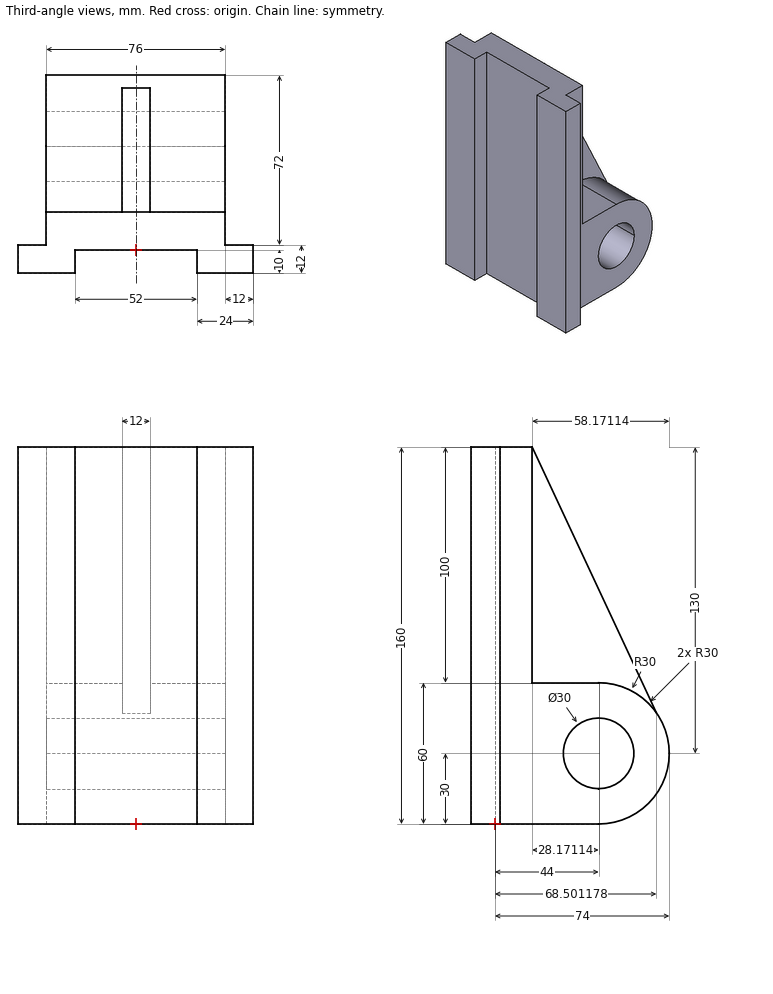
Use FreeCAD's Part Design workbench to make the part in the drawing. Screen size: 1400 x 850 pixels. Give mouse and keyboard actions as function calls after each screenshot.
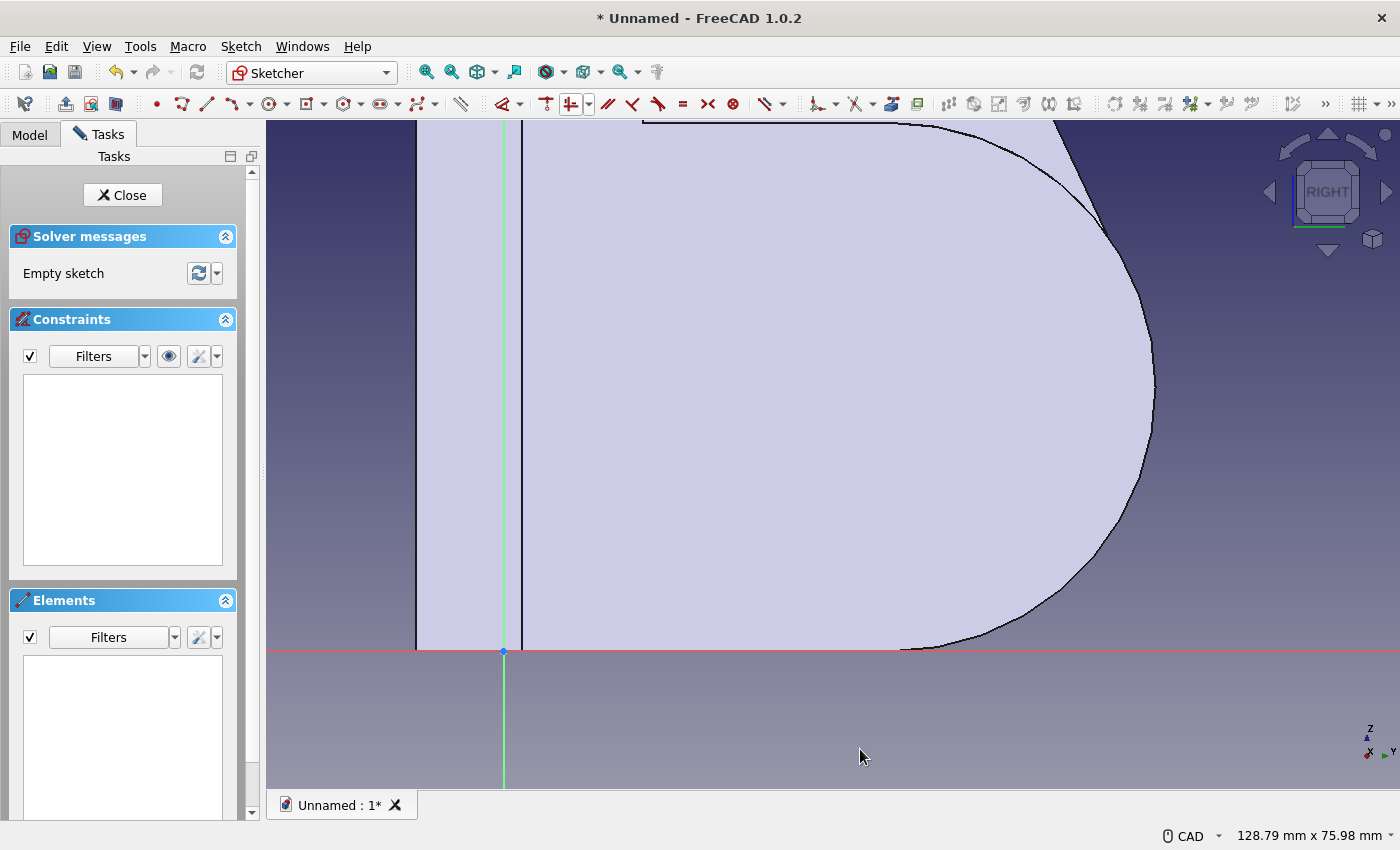
key(g)
key(c)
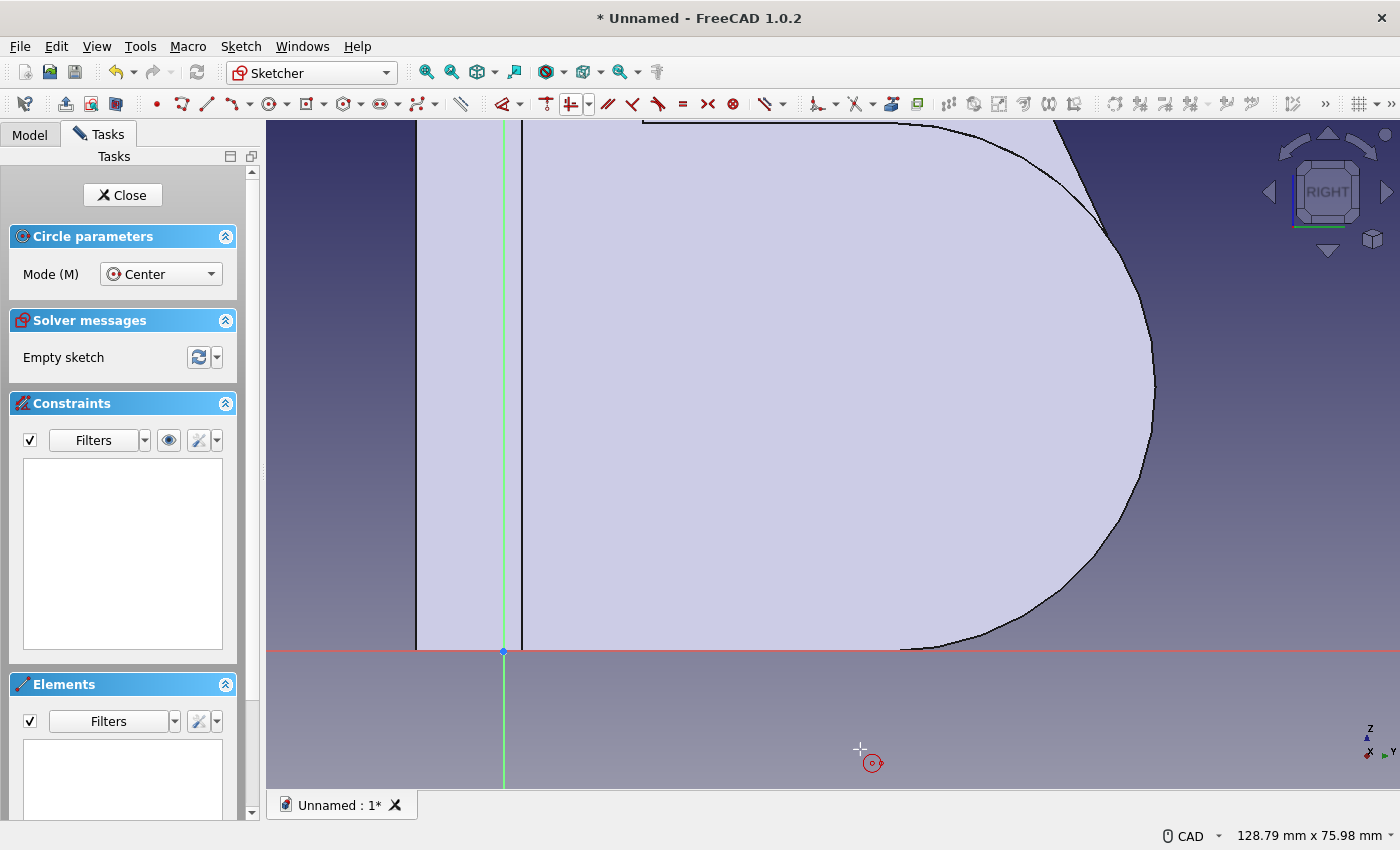
click(891, 387)
move(985, 294)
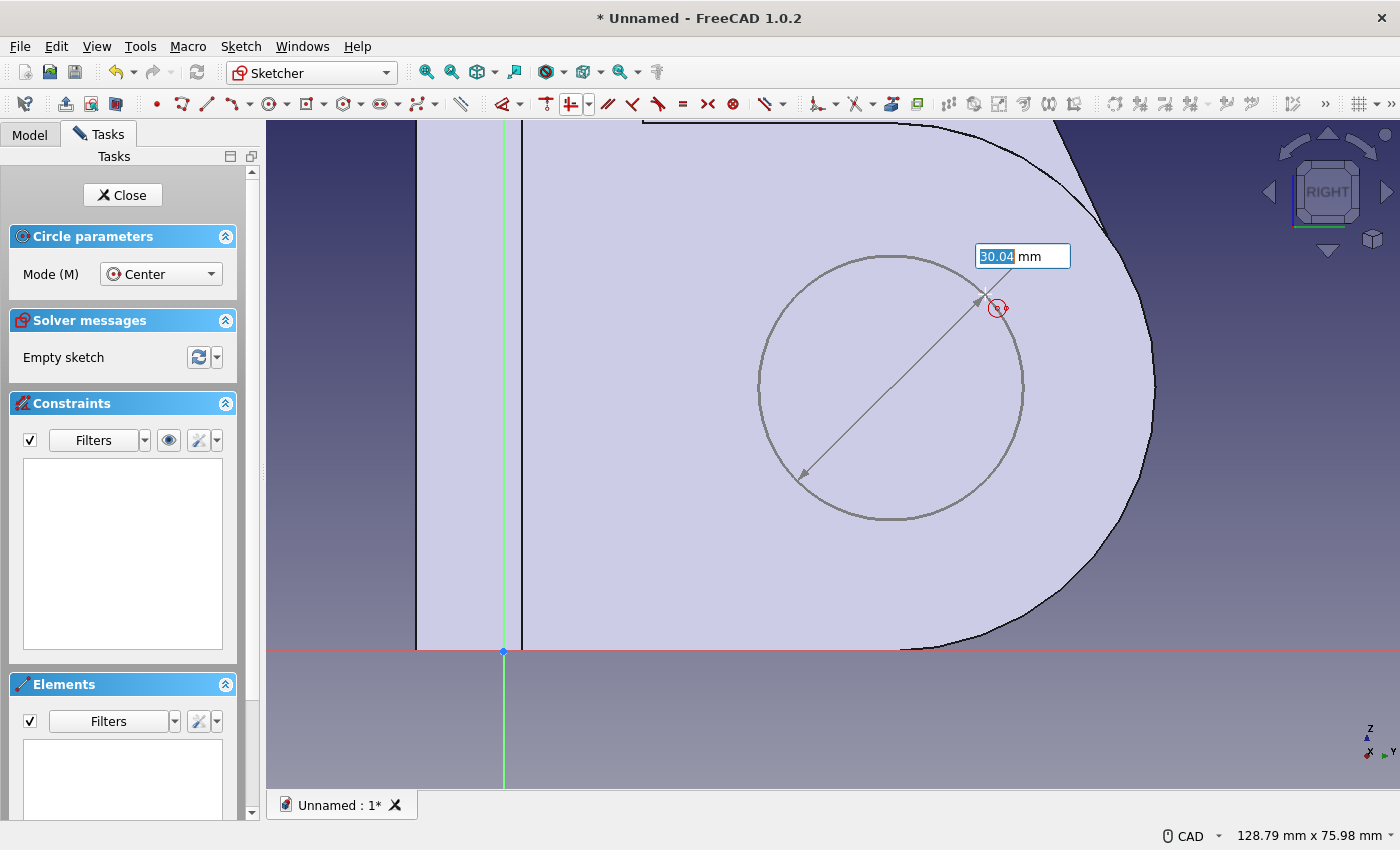
text(30)
key(Return)
key(Escape)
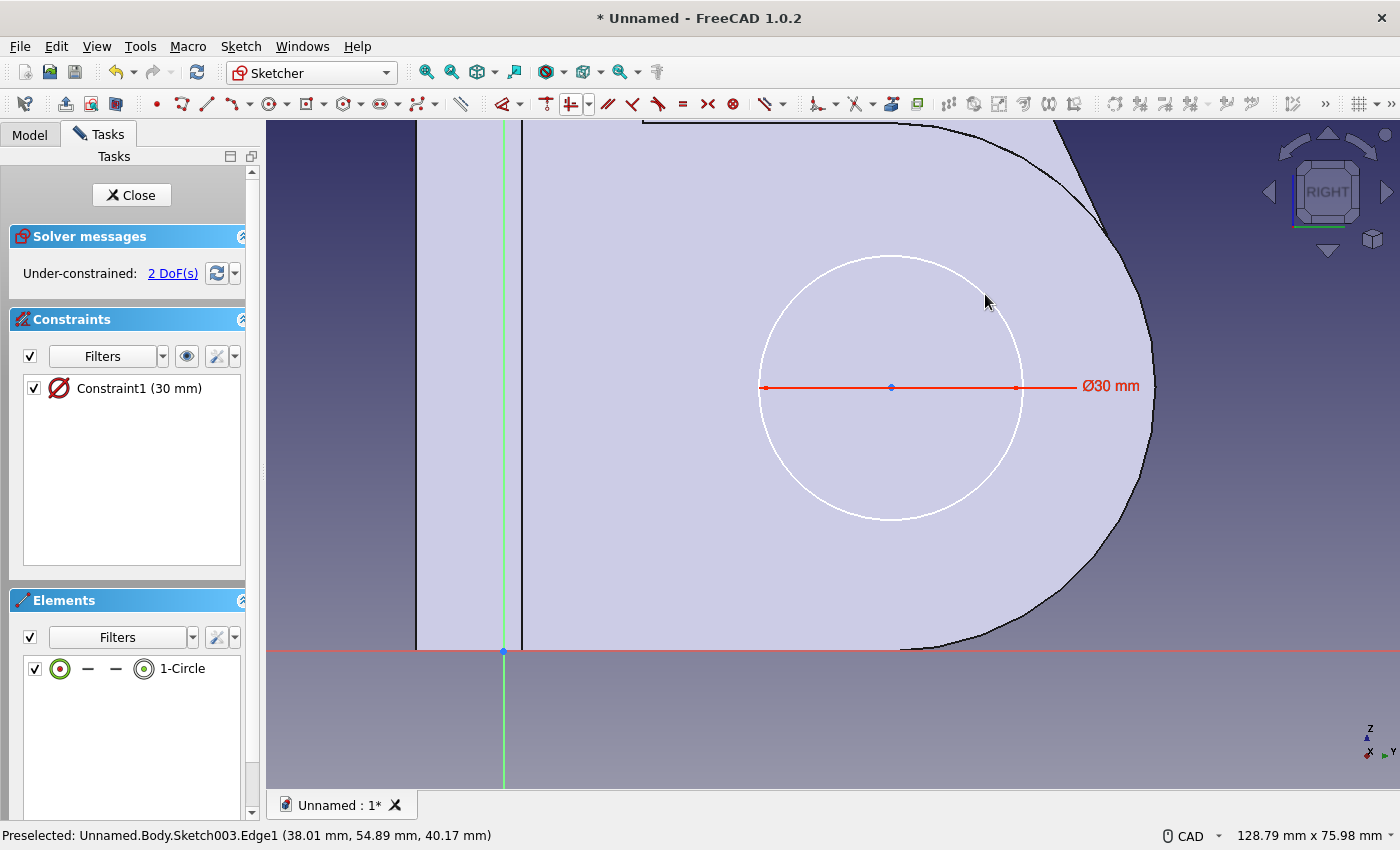
click(502, 104)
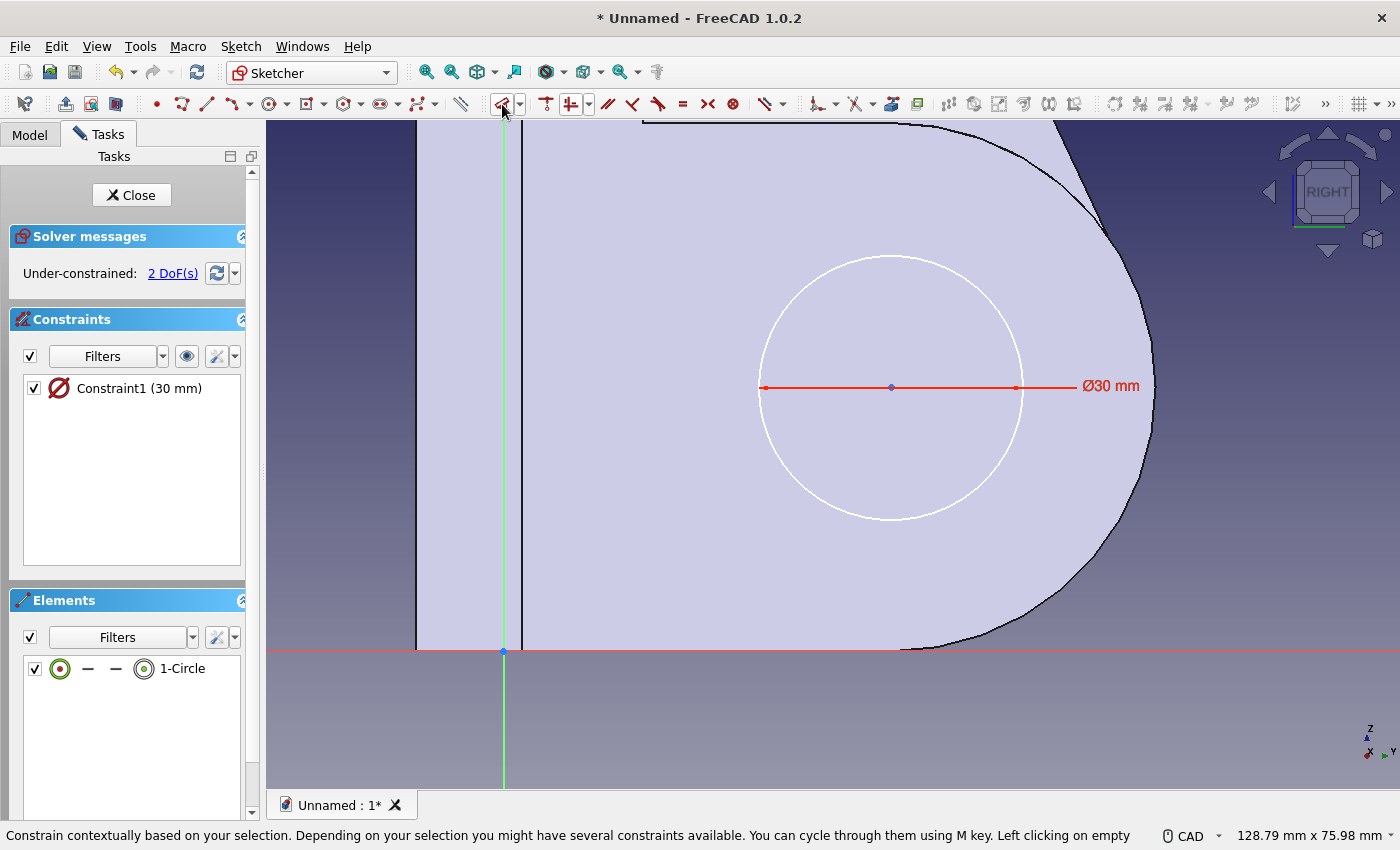
click(891, 388)
click(697, 685)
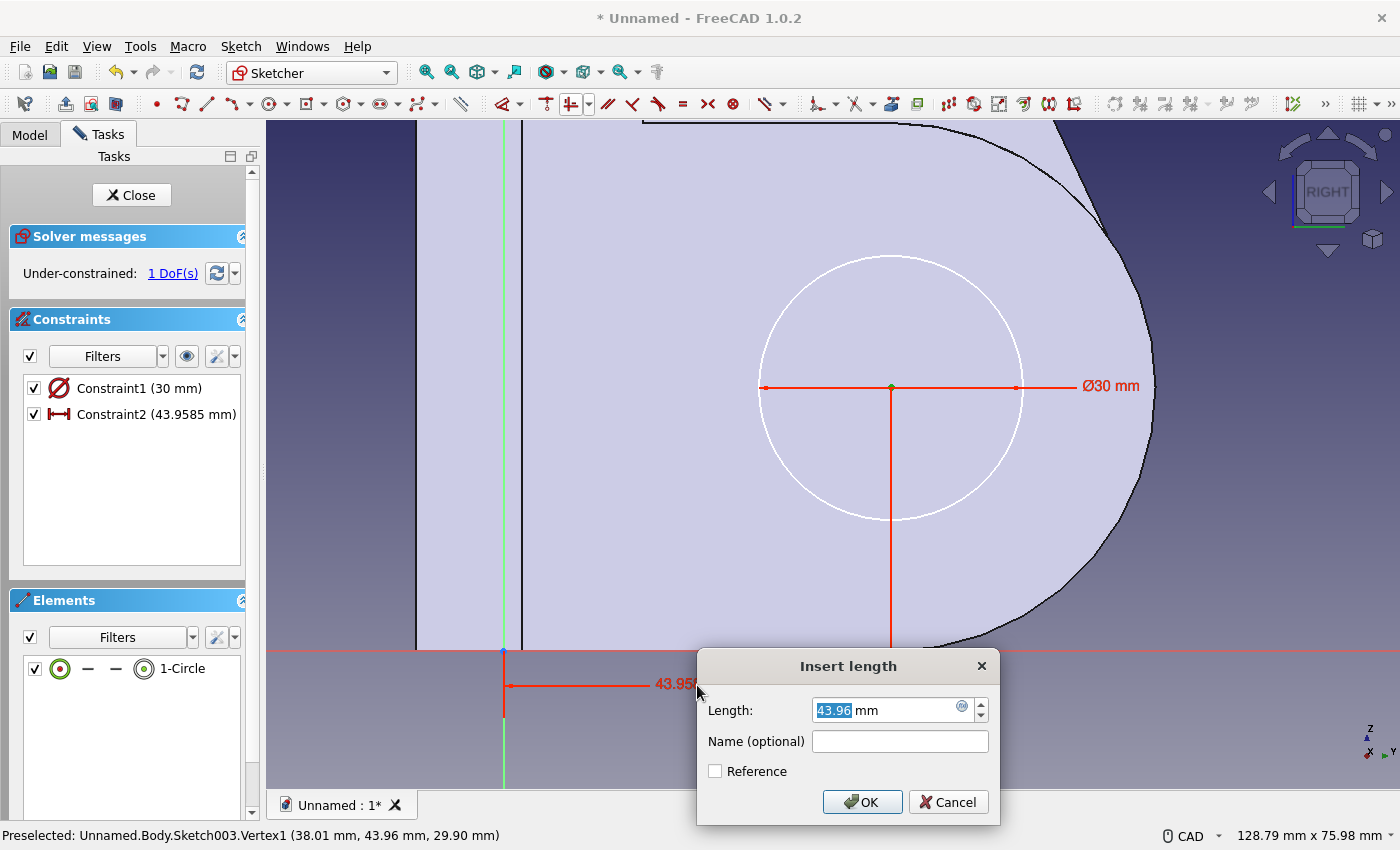
text(44)
key(Return)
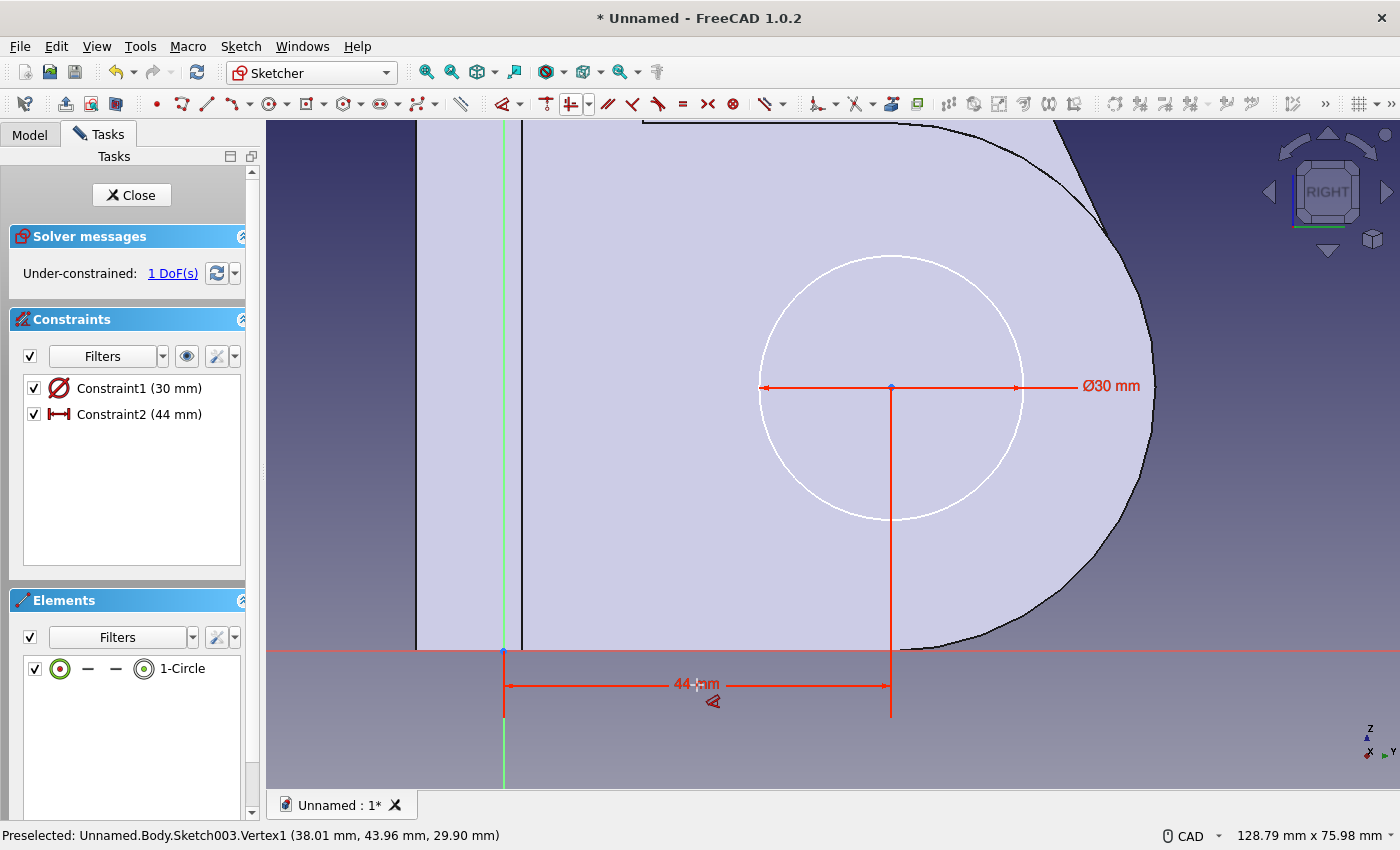
click(891, 388)
click(470, 520)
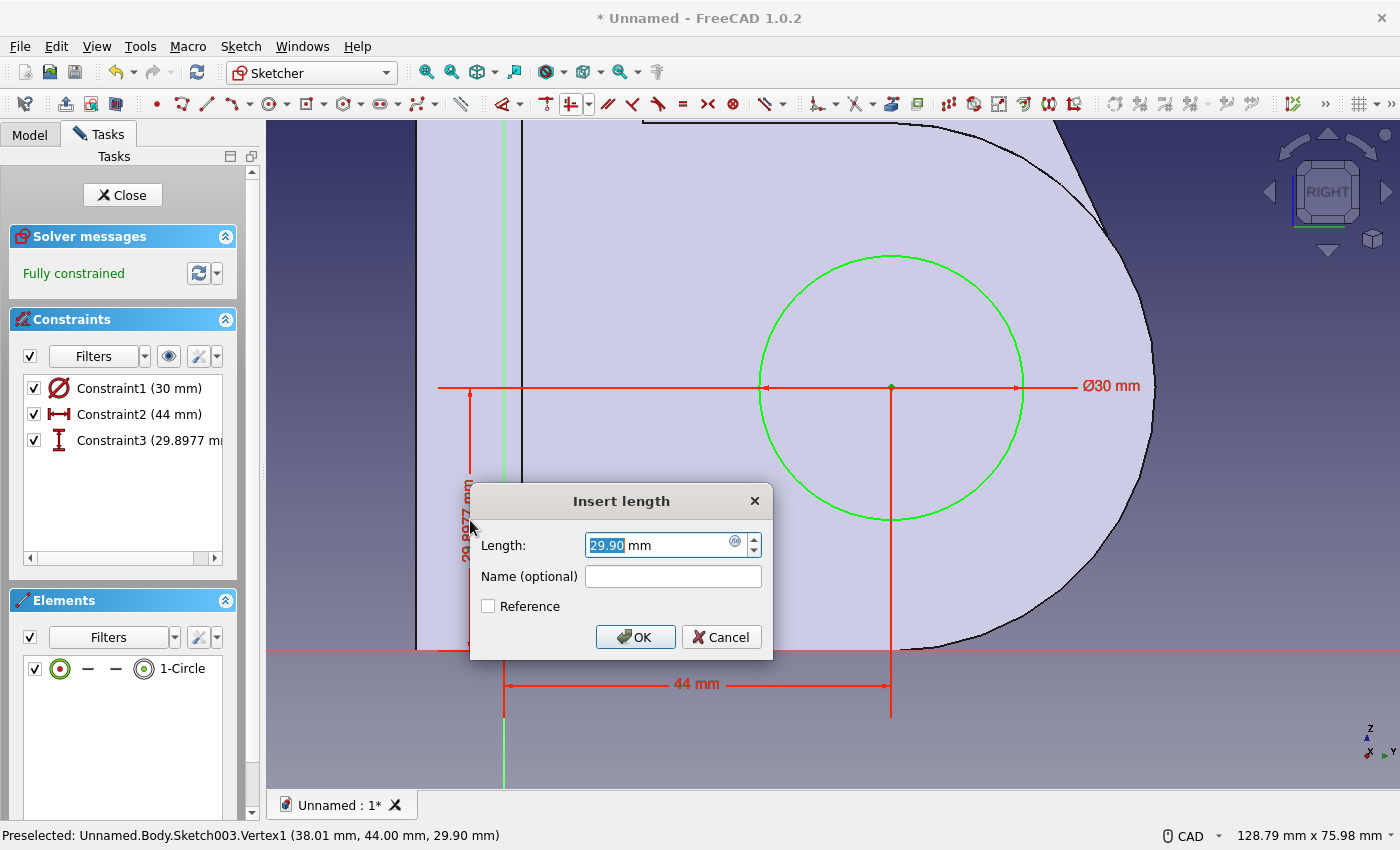
text(30)
key(Return)
key(Escape)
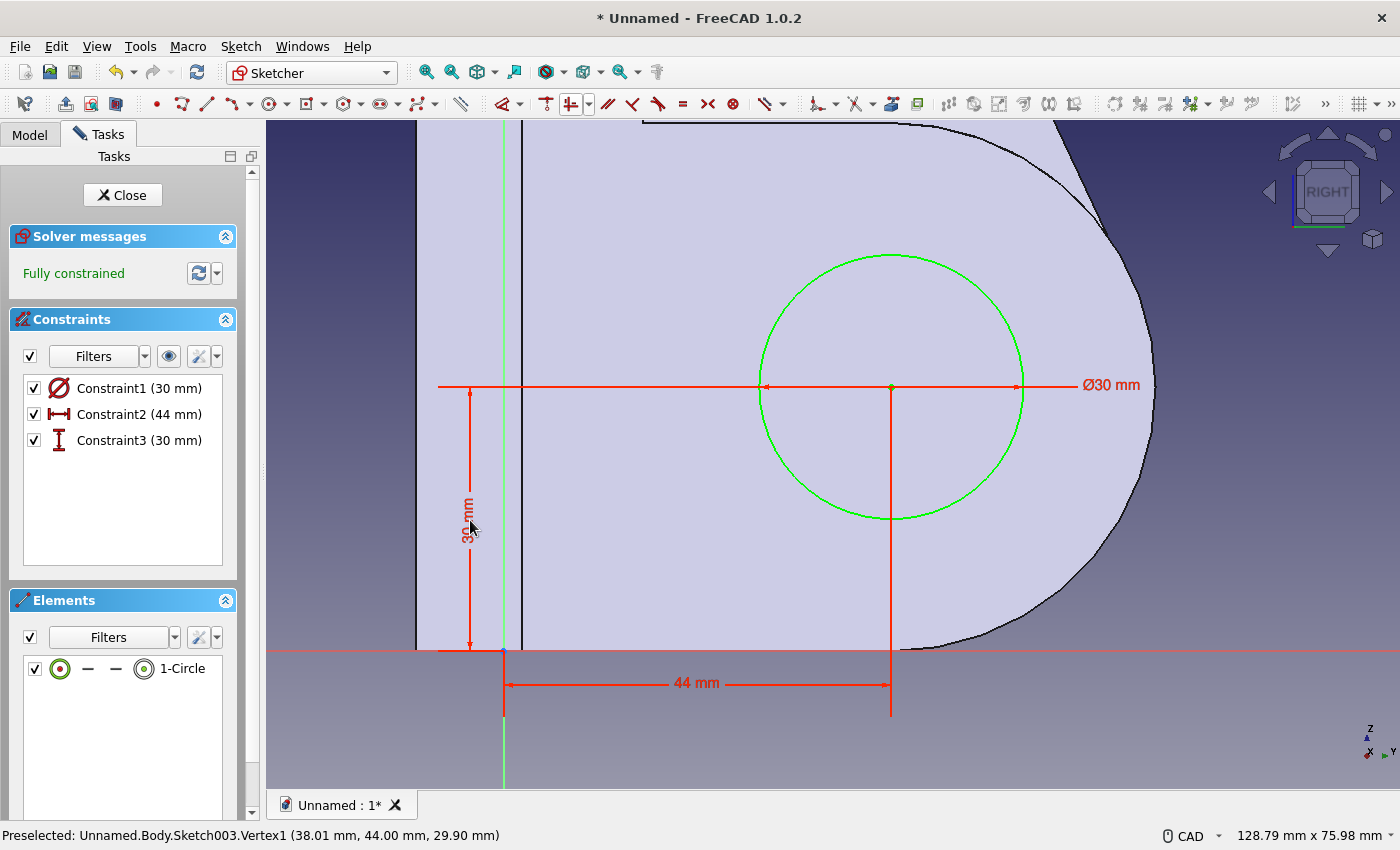
click(123, 195)